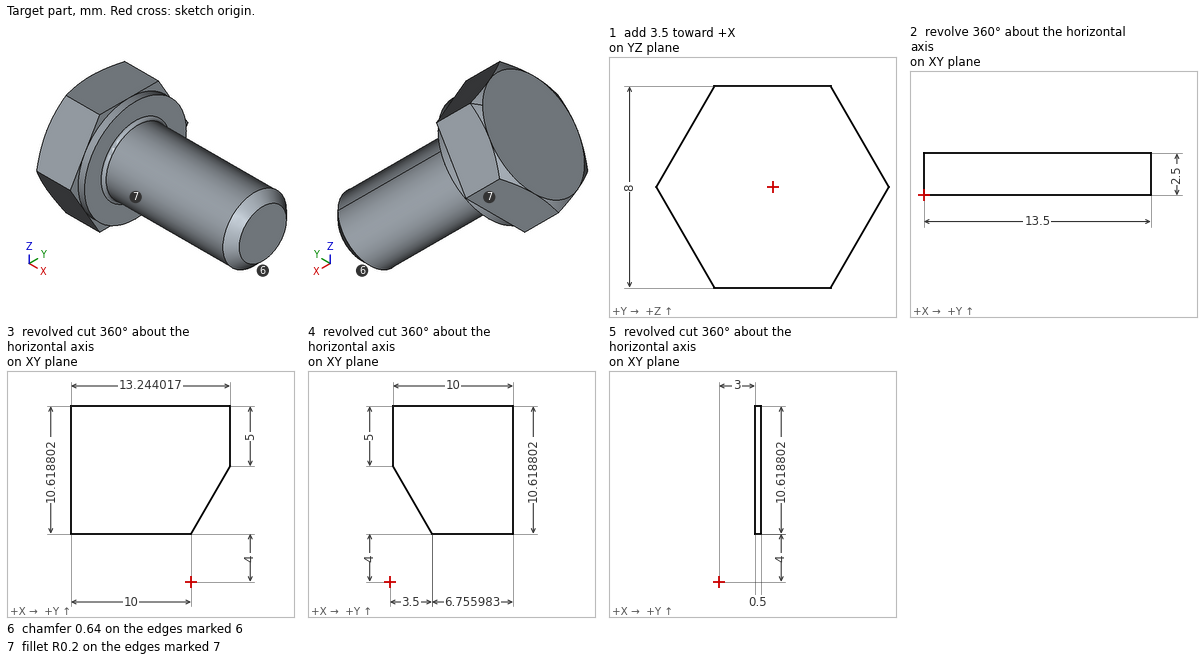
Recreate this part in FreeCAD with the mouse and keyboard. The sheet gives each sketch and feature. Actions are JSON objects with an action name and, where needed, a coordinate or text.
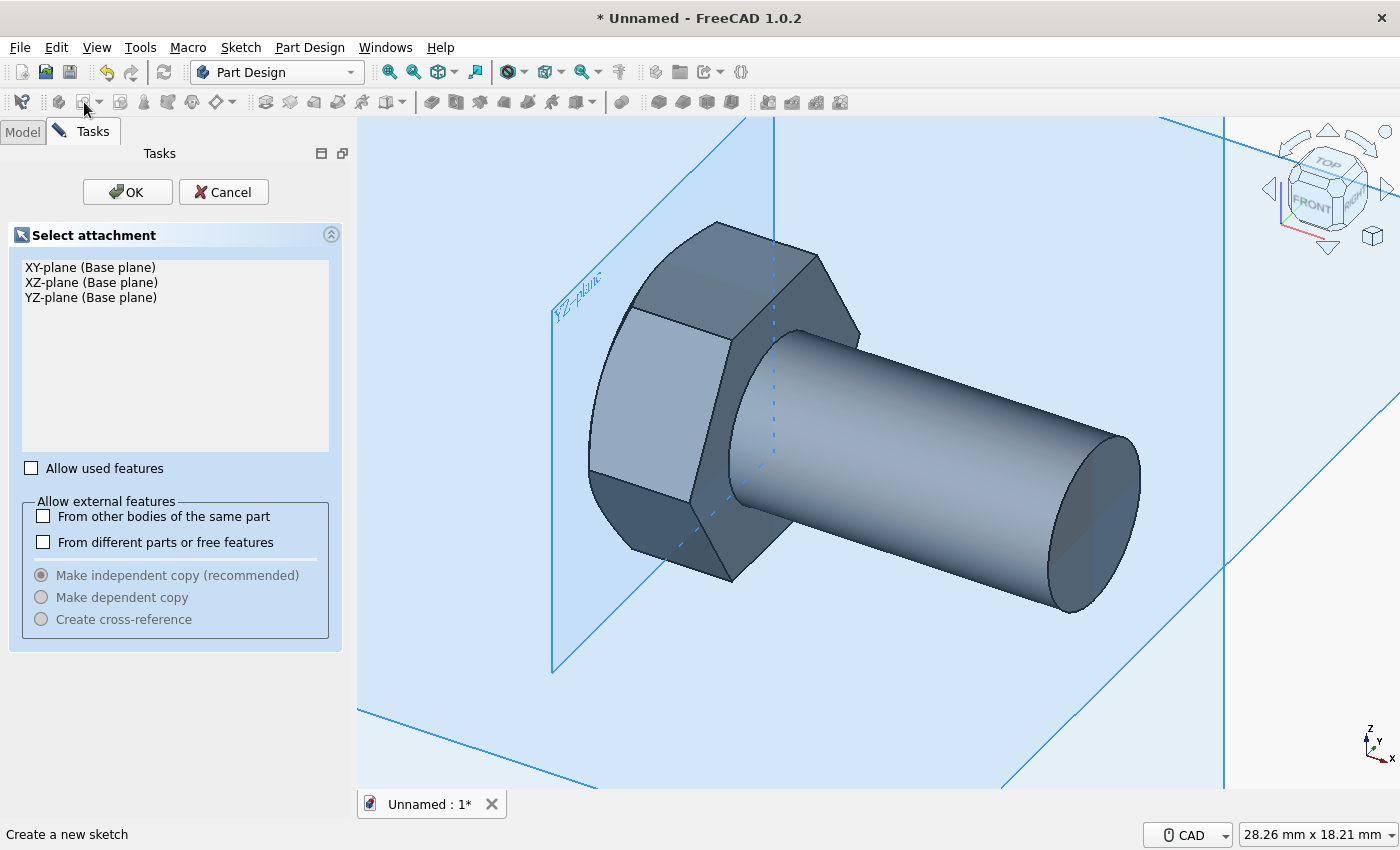
{"action": "left_click", "coordinate": [82, 268]}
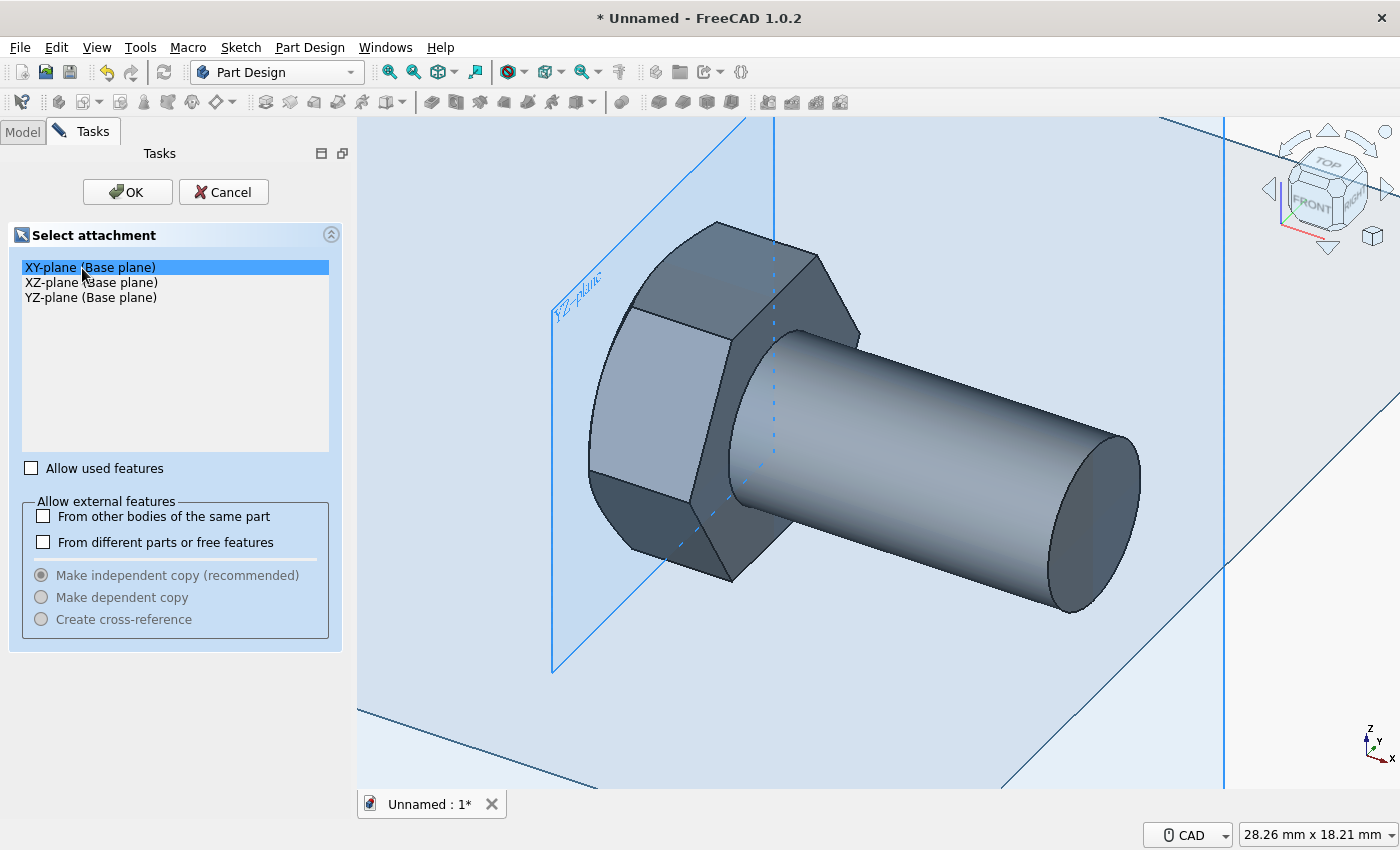
{"action": "left_click", "coordinate": [128, 192]}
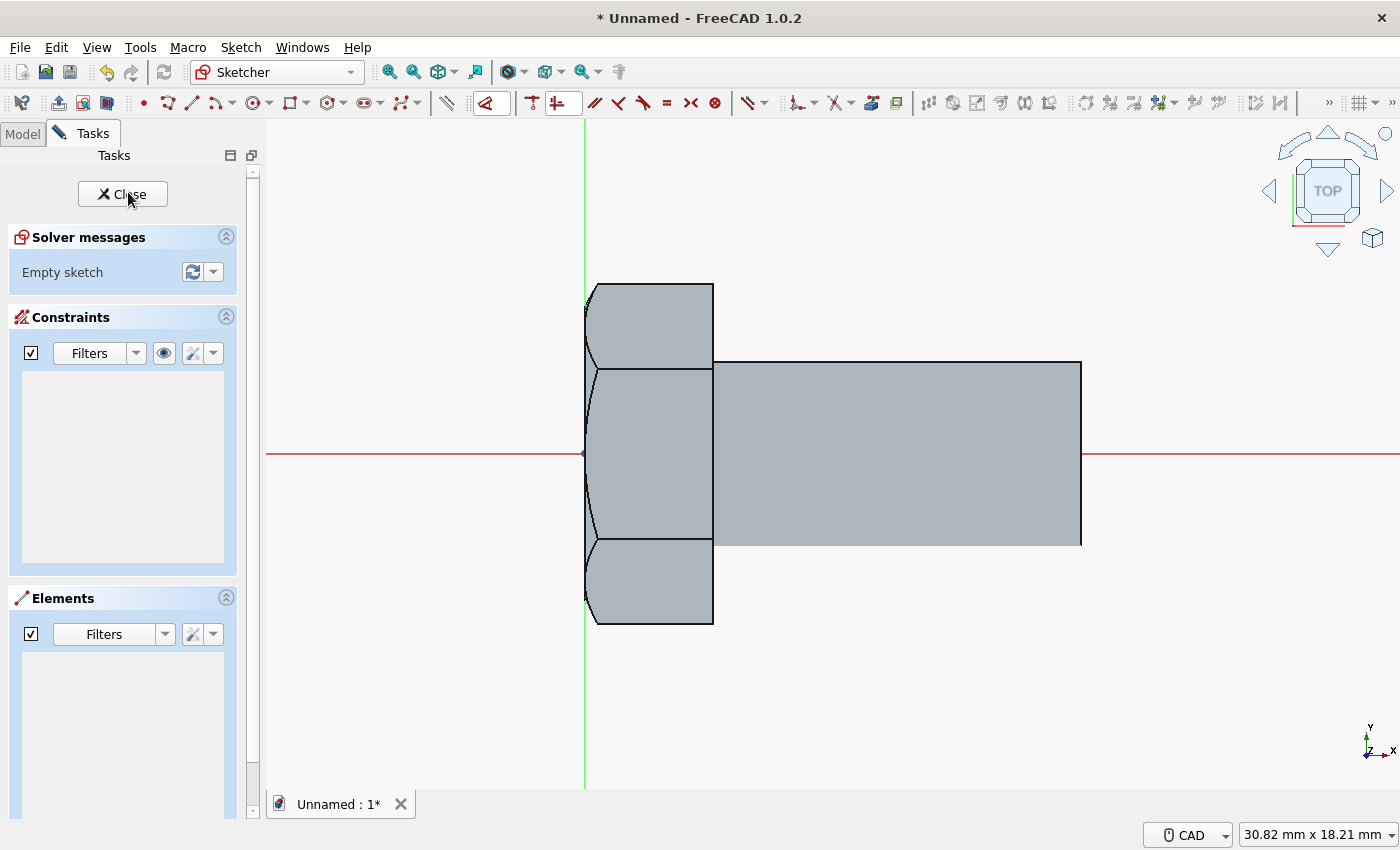
{"action": "left_click", "coordinate": [108, 104]}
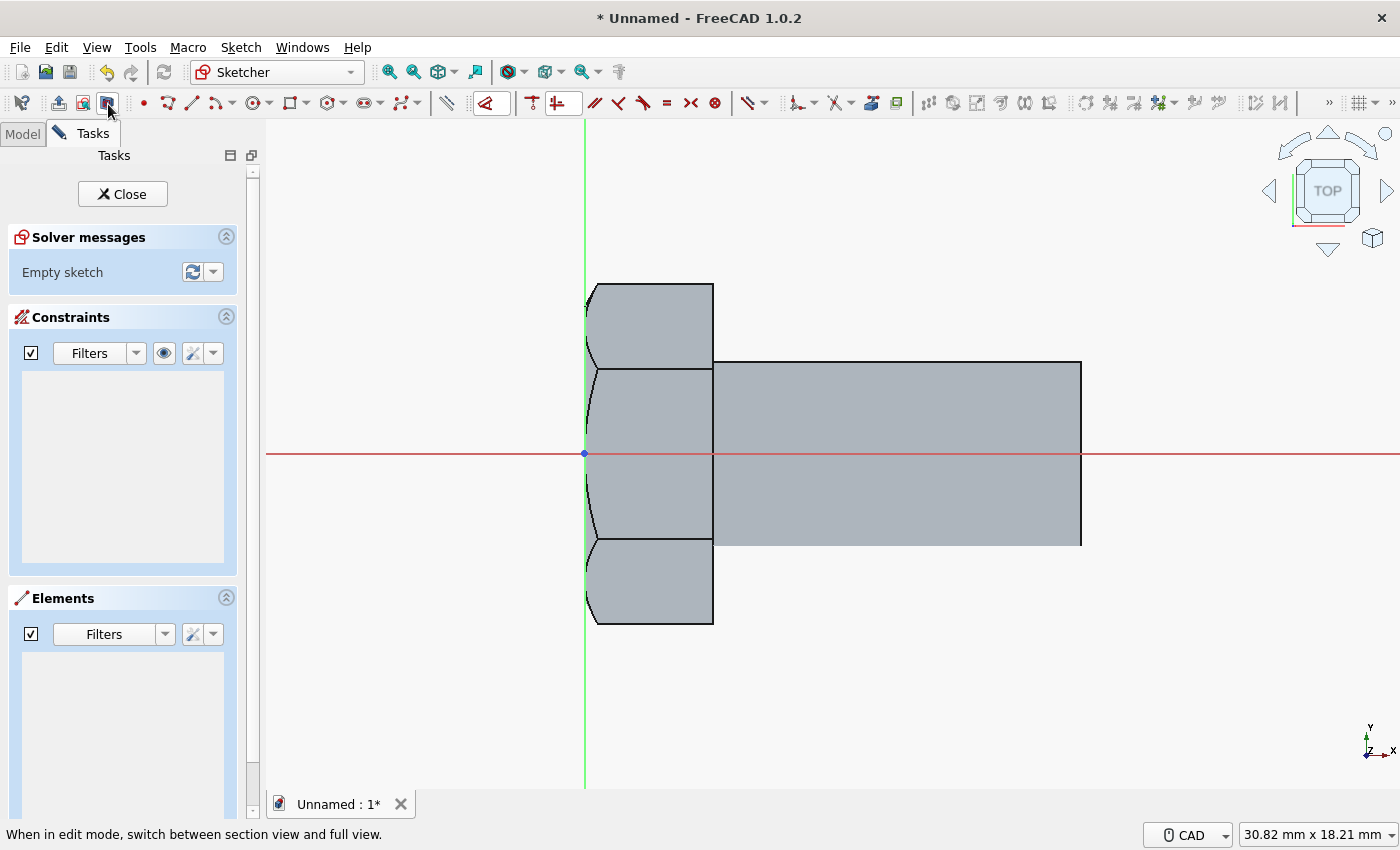
{"action": "scroll", "coordinate": [747, 761], "scroll_direction": "down", "scroll_amount": 2}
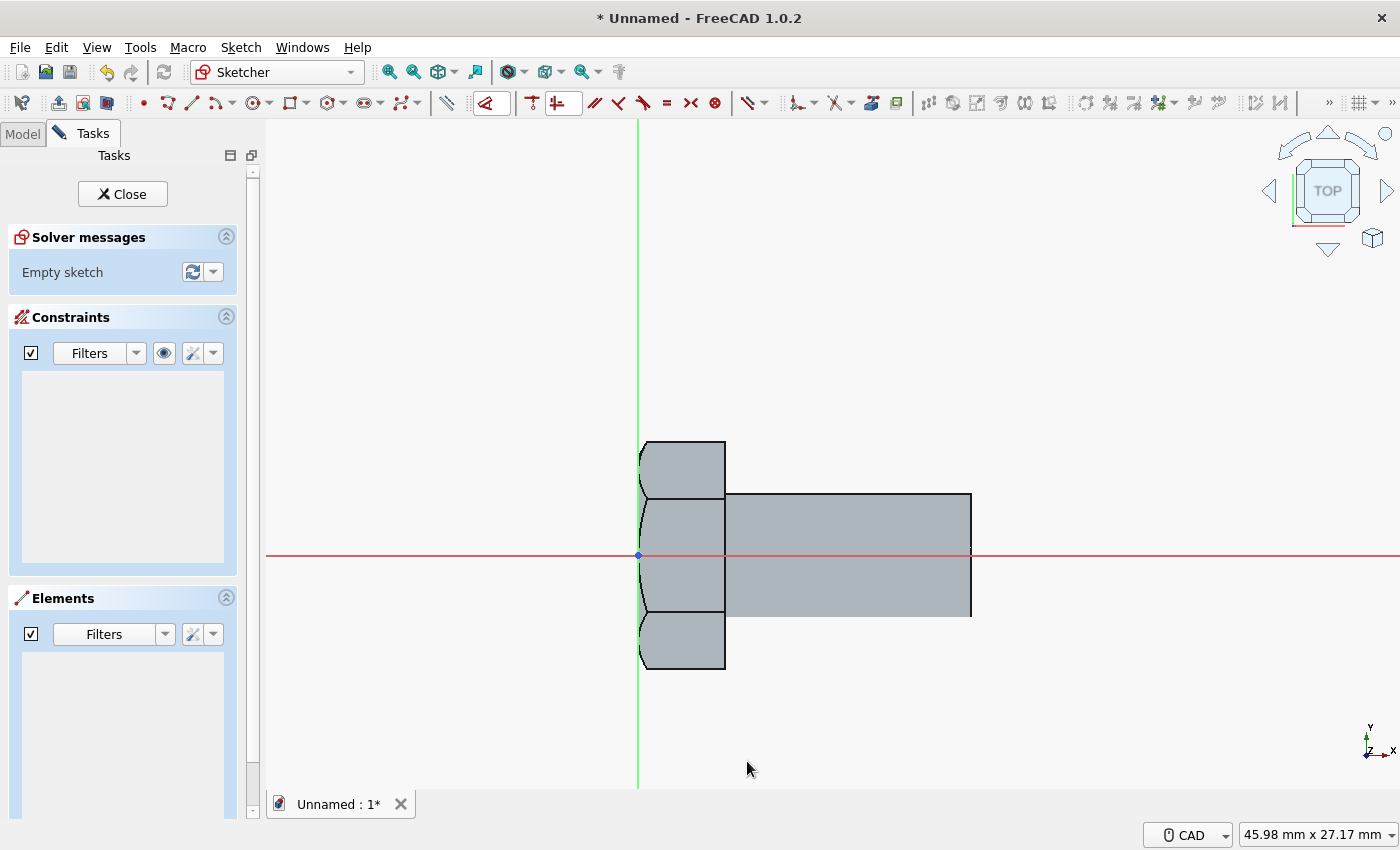
{"action": "left_click", "coordinate": [168, 104]}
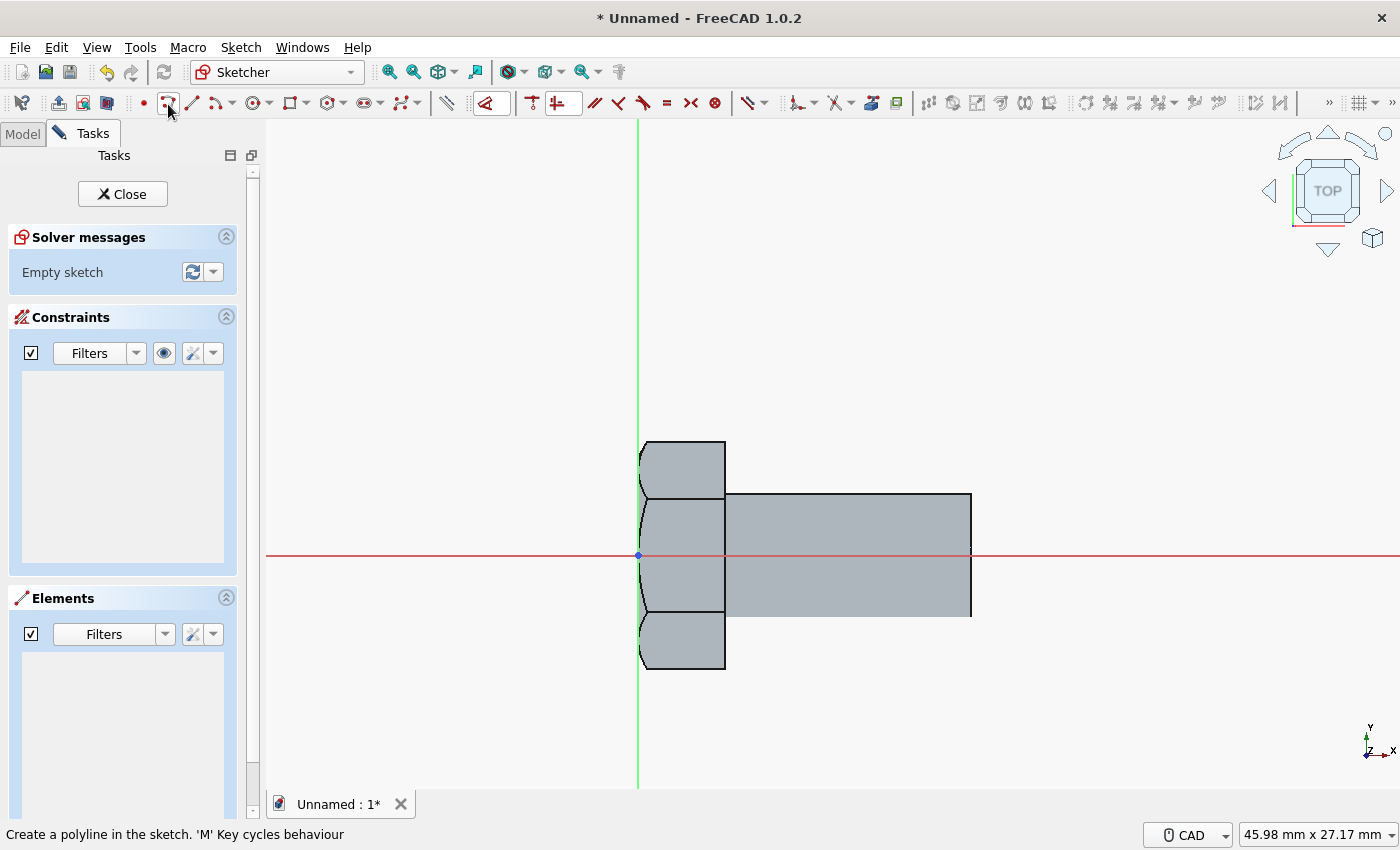
{"action": "left_click", "coordinate": [725, 457]}
{"action": "left_click", "coordinate": [891, 457]}
{"action": "left_click", "coordinate": [891, 195]}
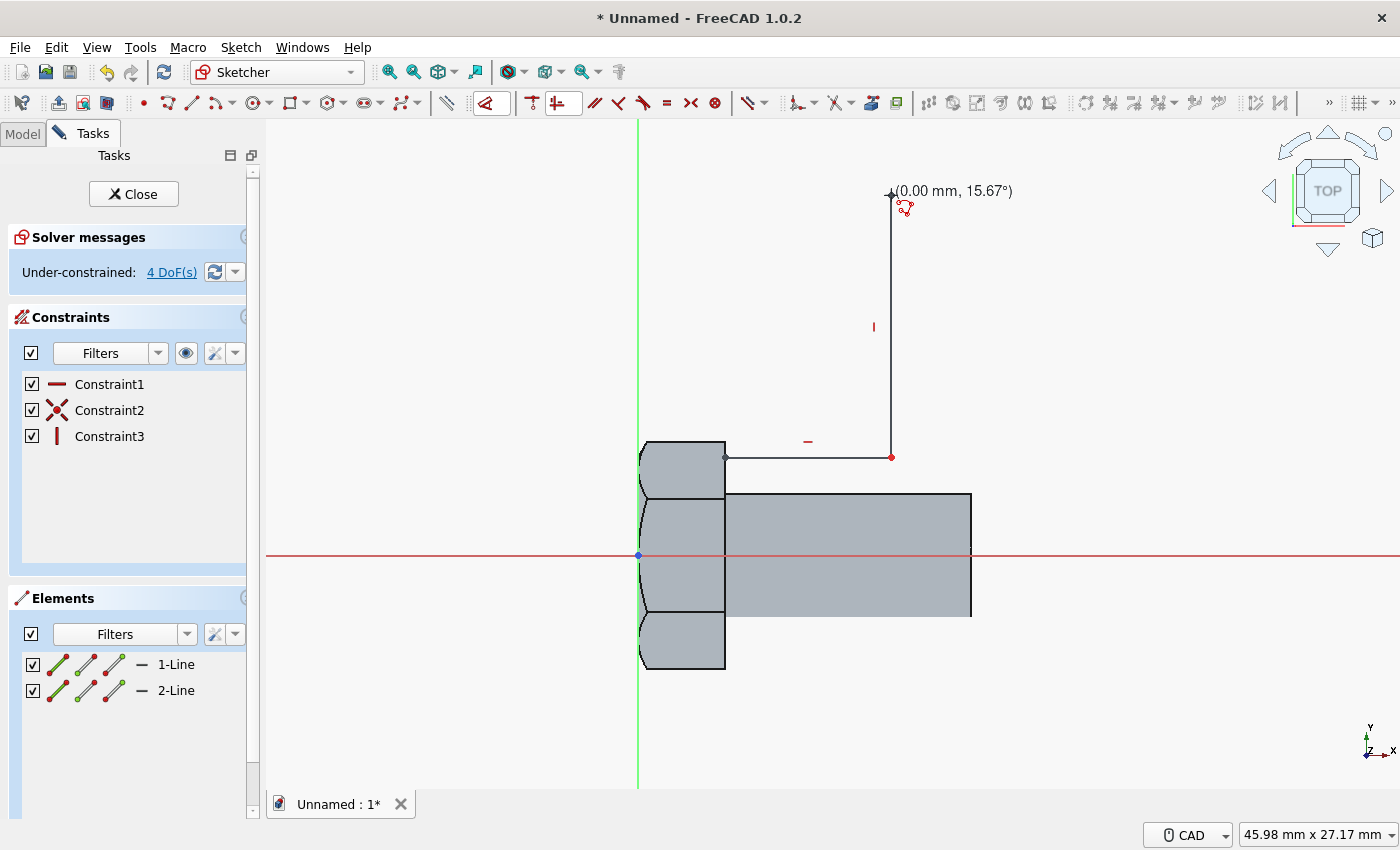
{"action": "scroll", "coordinate": [645, 195], "scroll_direction": "up", "scroll_amount": 5}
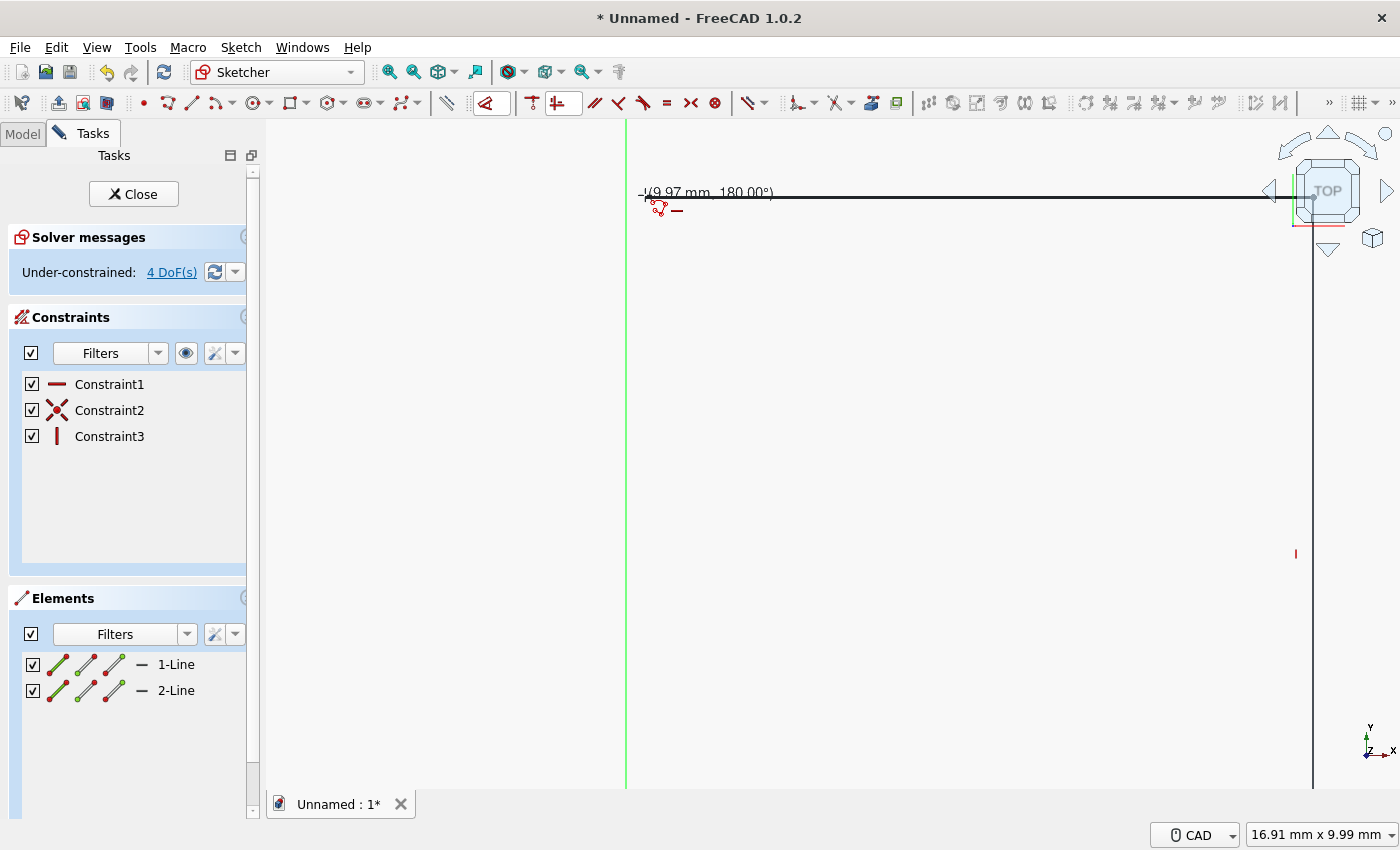
{"action": "left_click", "coordinate": [643, 195]}
{"action": "left_click", "coordinate": [643, 530]}